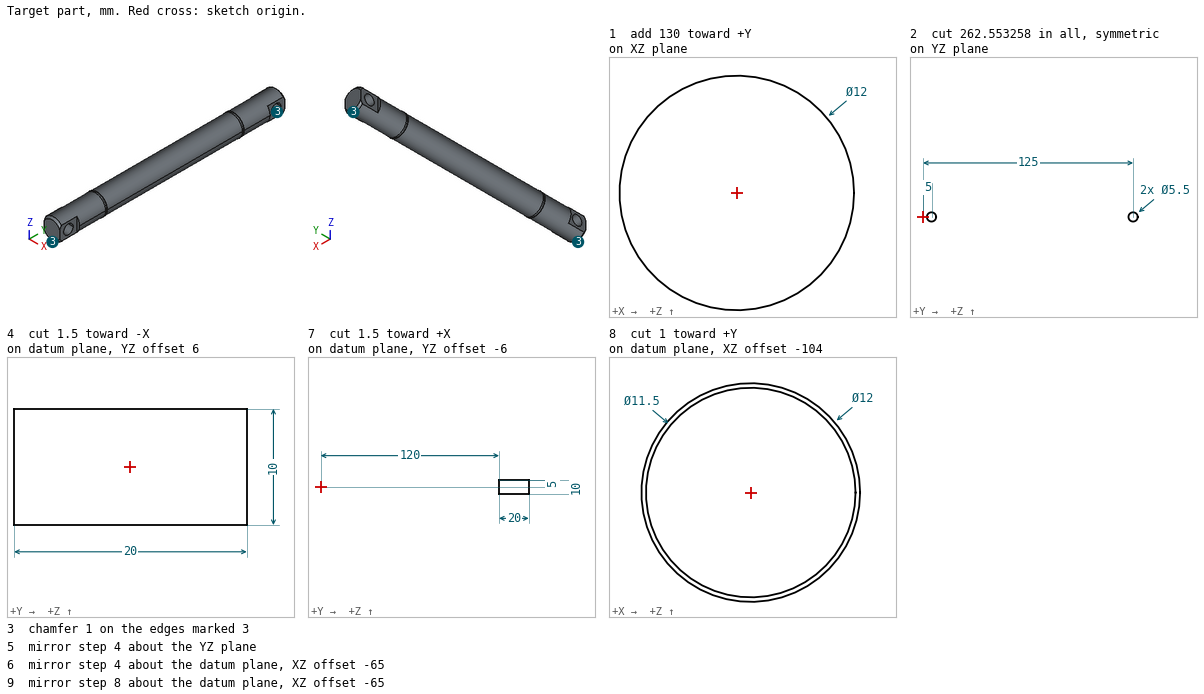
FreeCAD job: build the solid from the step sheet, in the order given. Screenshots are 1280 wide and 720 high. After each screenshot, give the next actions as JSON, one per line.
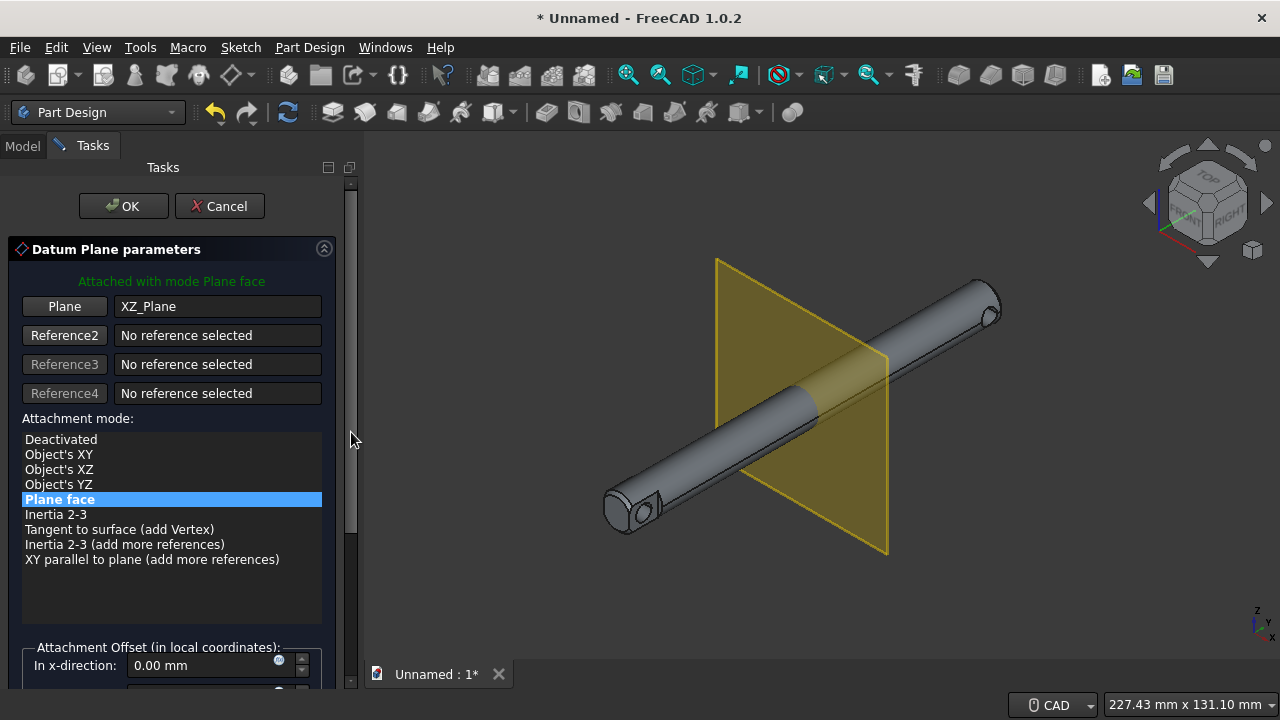
{"action": "left_click", "coordinate": [124, 206]}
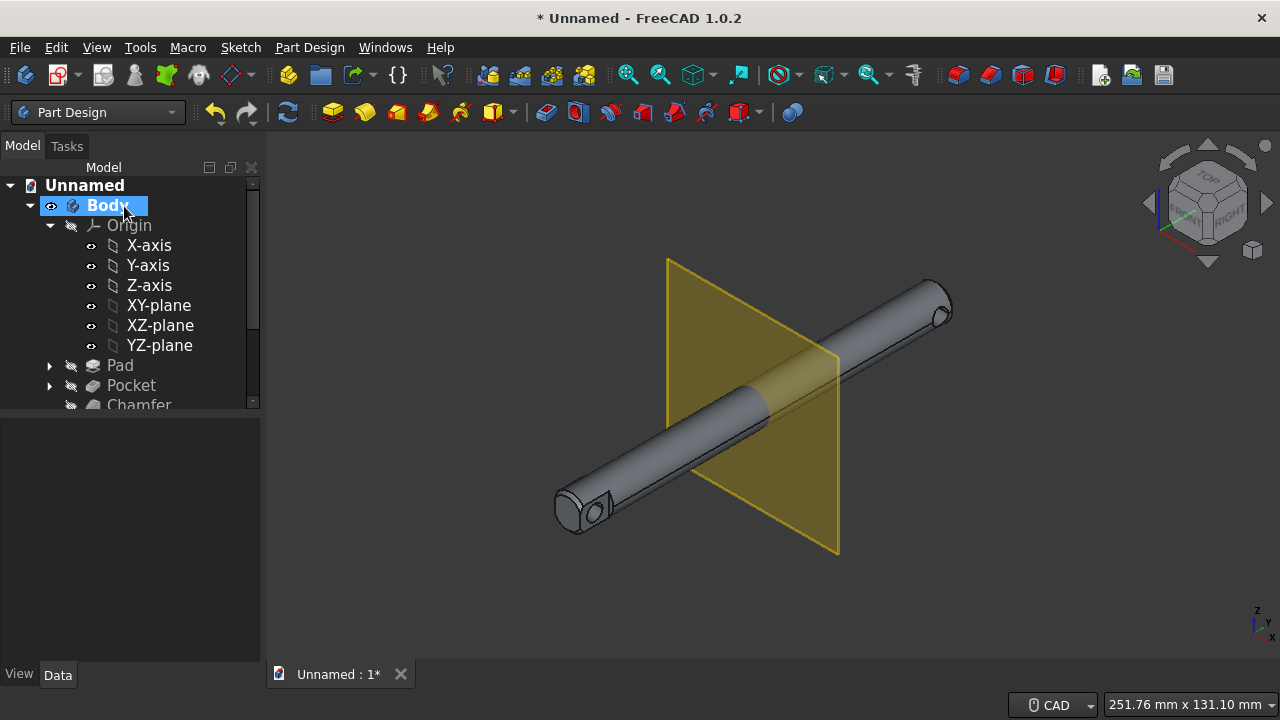
{"action": "scroll", "coordinate": [100, 301], "scroll_direction": "down", "scroll_amount": 3}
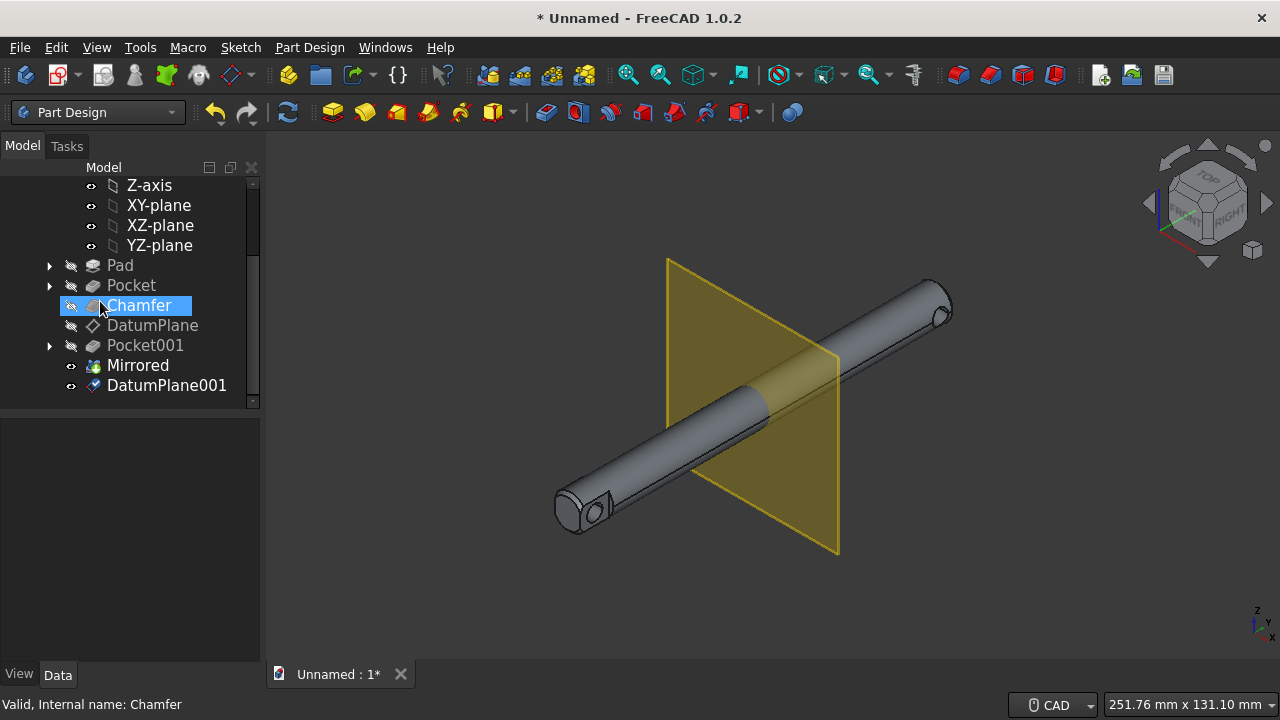
{"action": "left_click", "coordinate": [116, 346]}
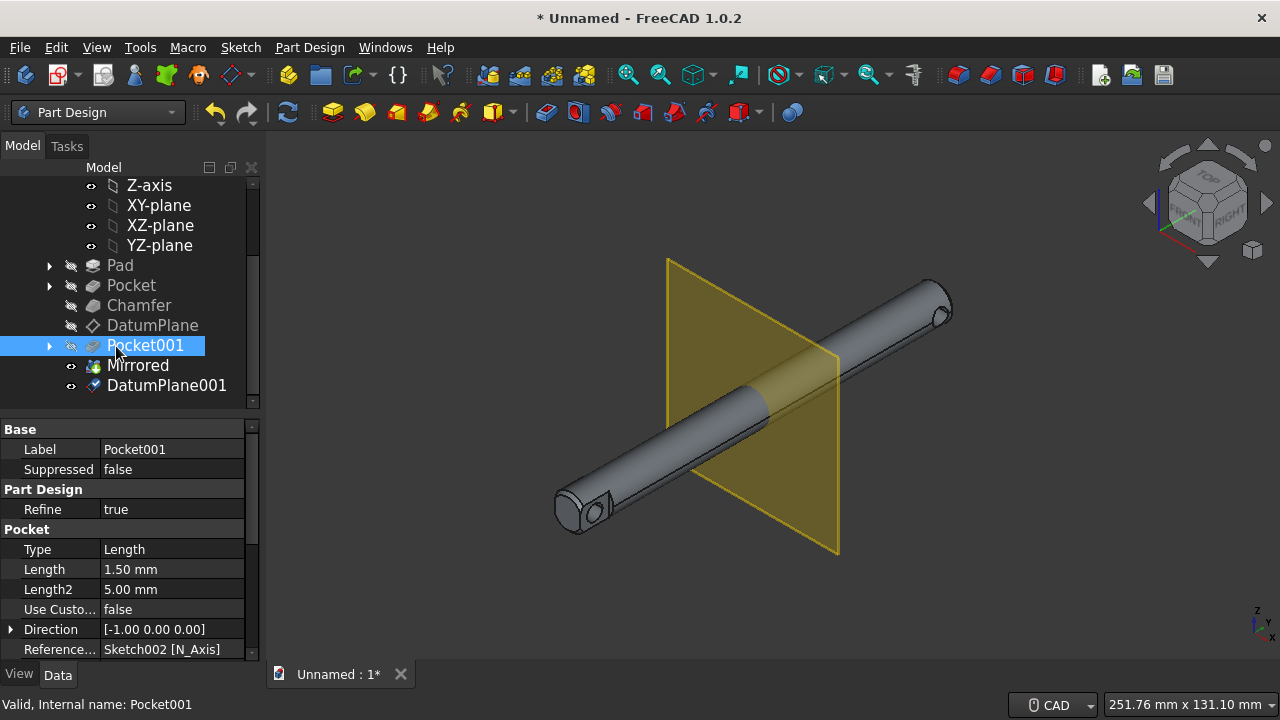
{"action": "left_click", "coordinate": [488, 76]}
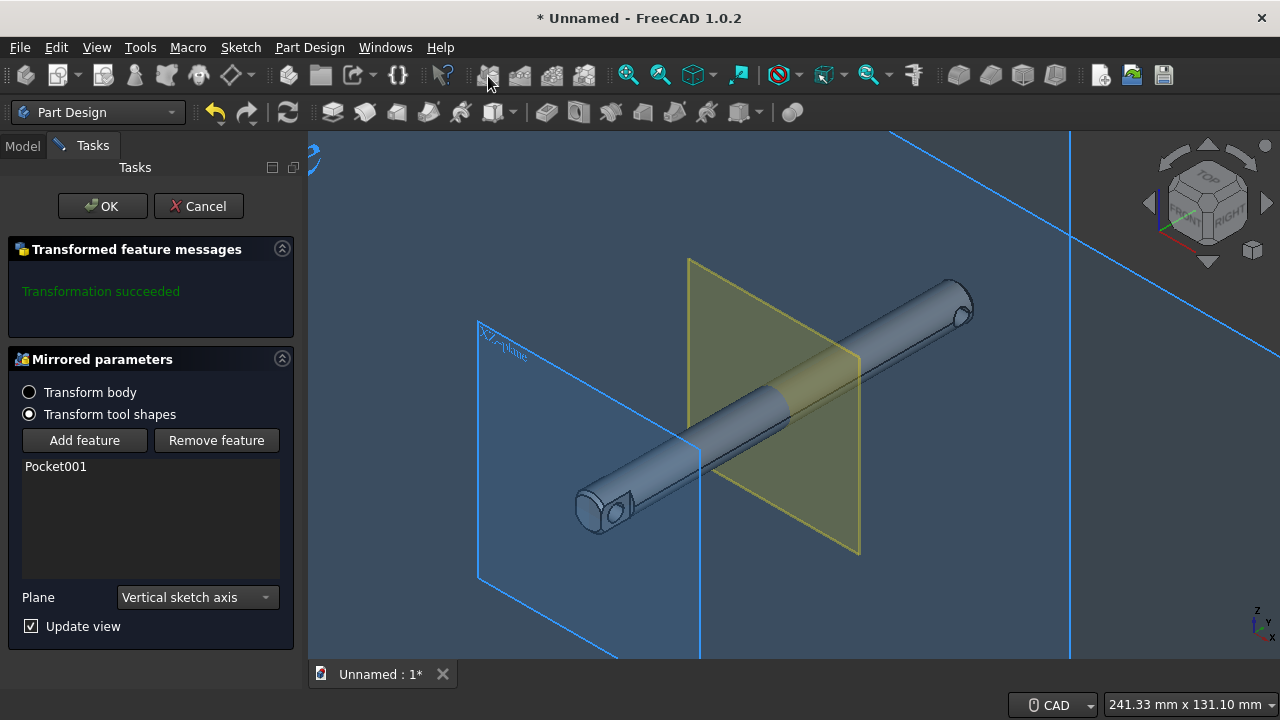
{"action": "left_click", "coordinate": [198, 598]}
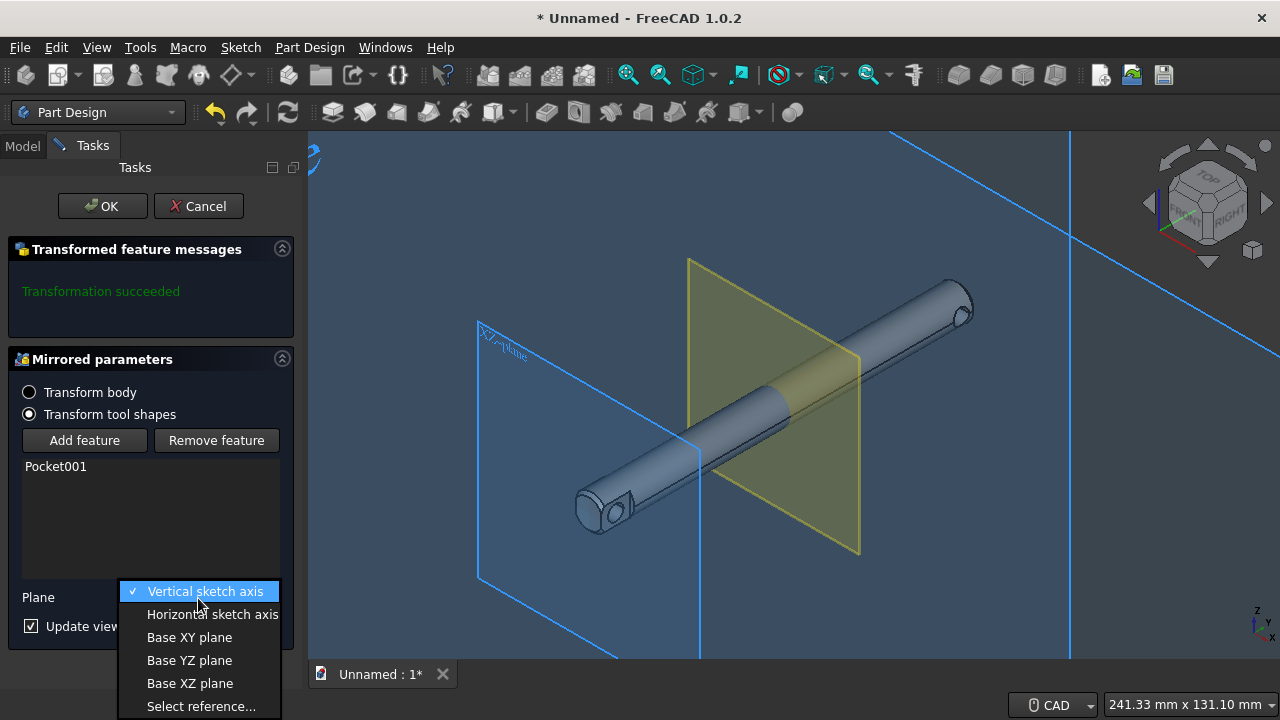
{"action": "left_click", "coordinate": [198, 706]}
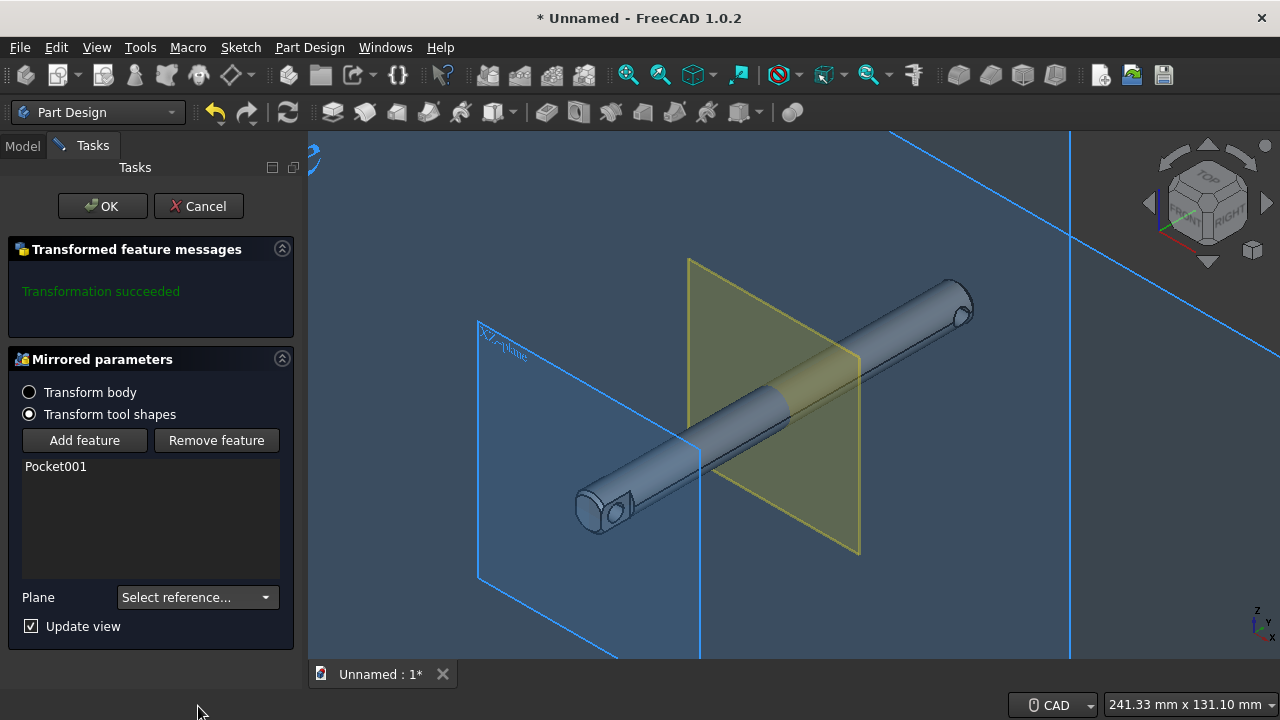
{"action": "left_click", "coordinate": [23, 145]}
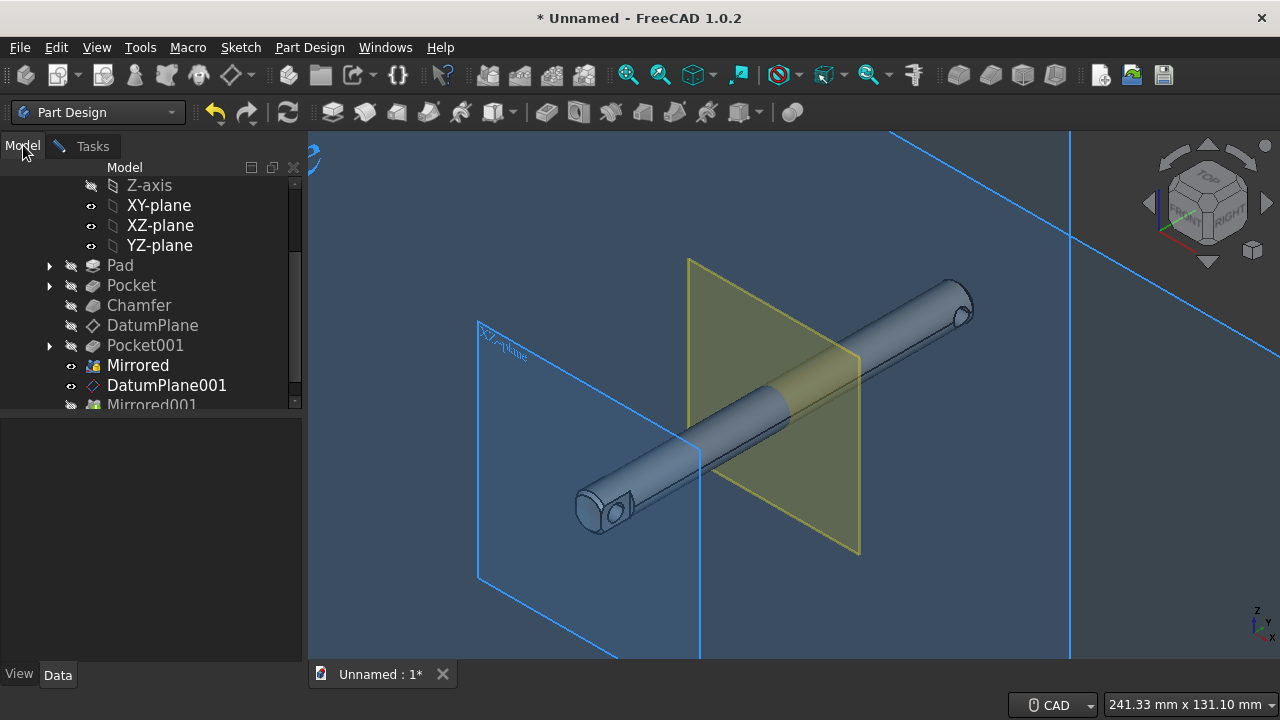
{"action": "left_click", "coordinate": [116, 386]}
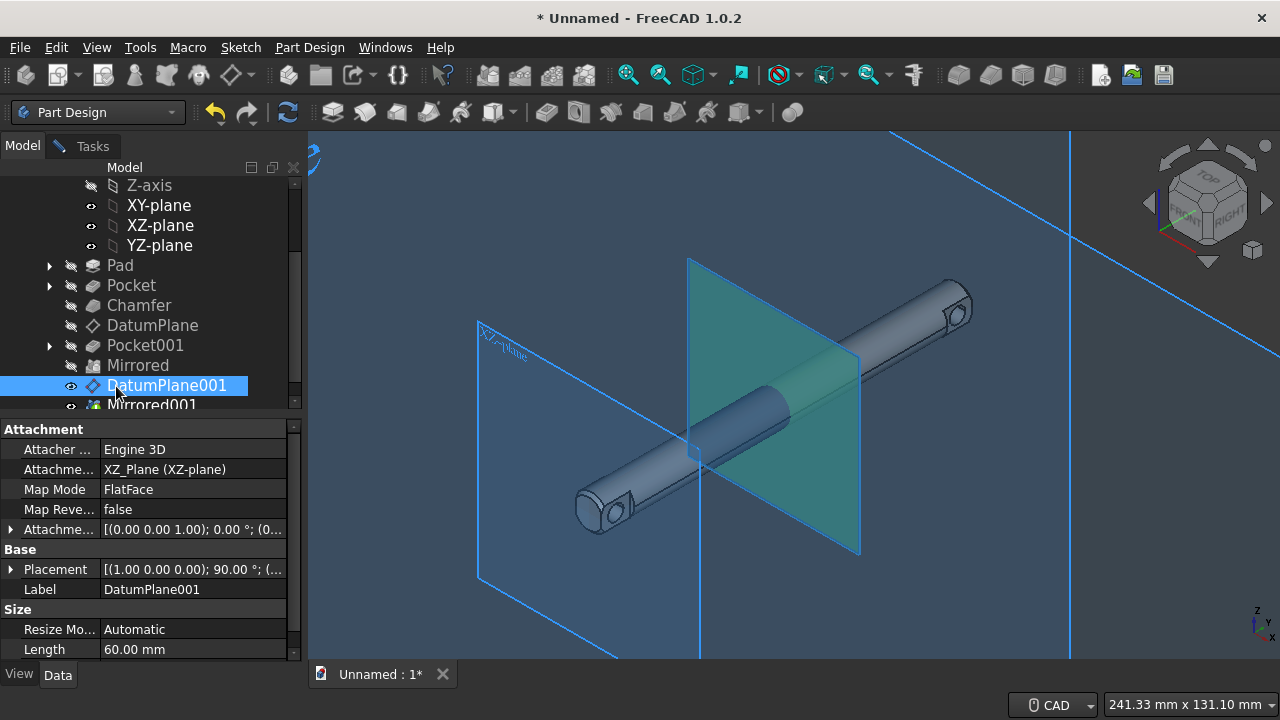
{"action": "left_click", "coordinate": [84, 145]}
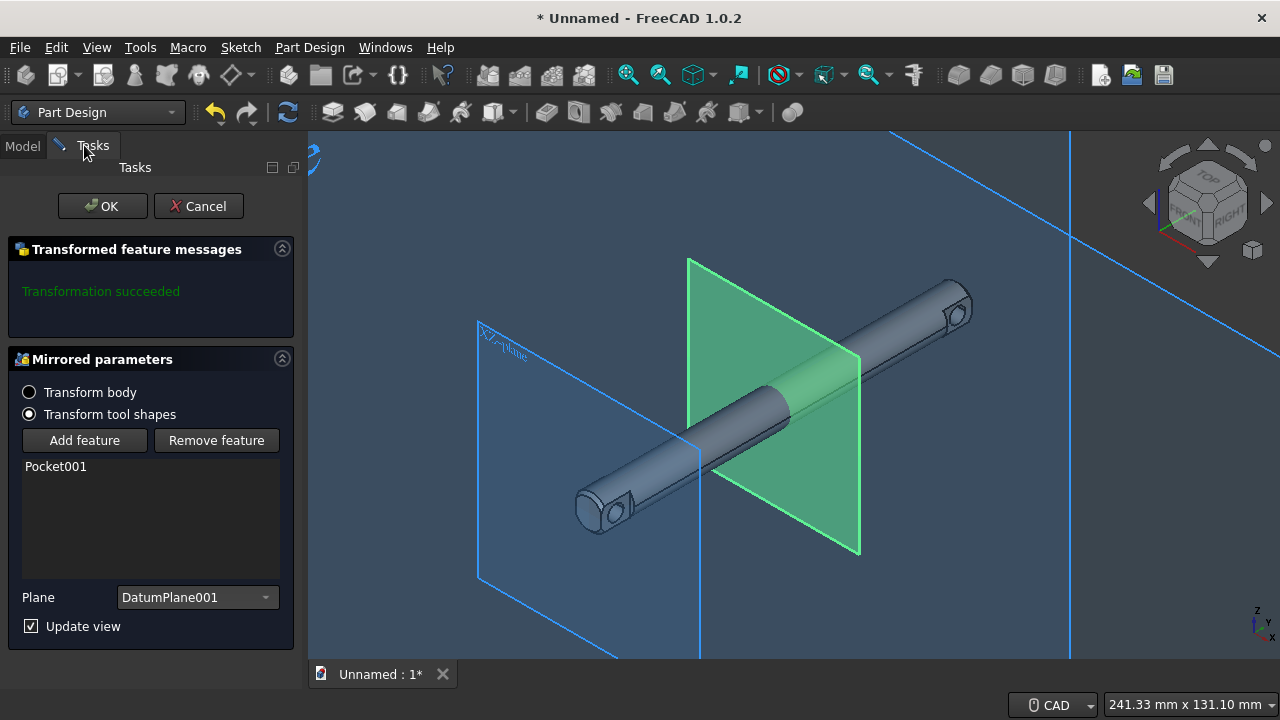
{"action": "left_click", "coordinate": [103, 206]}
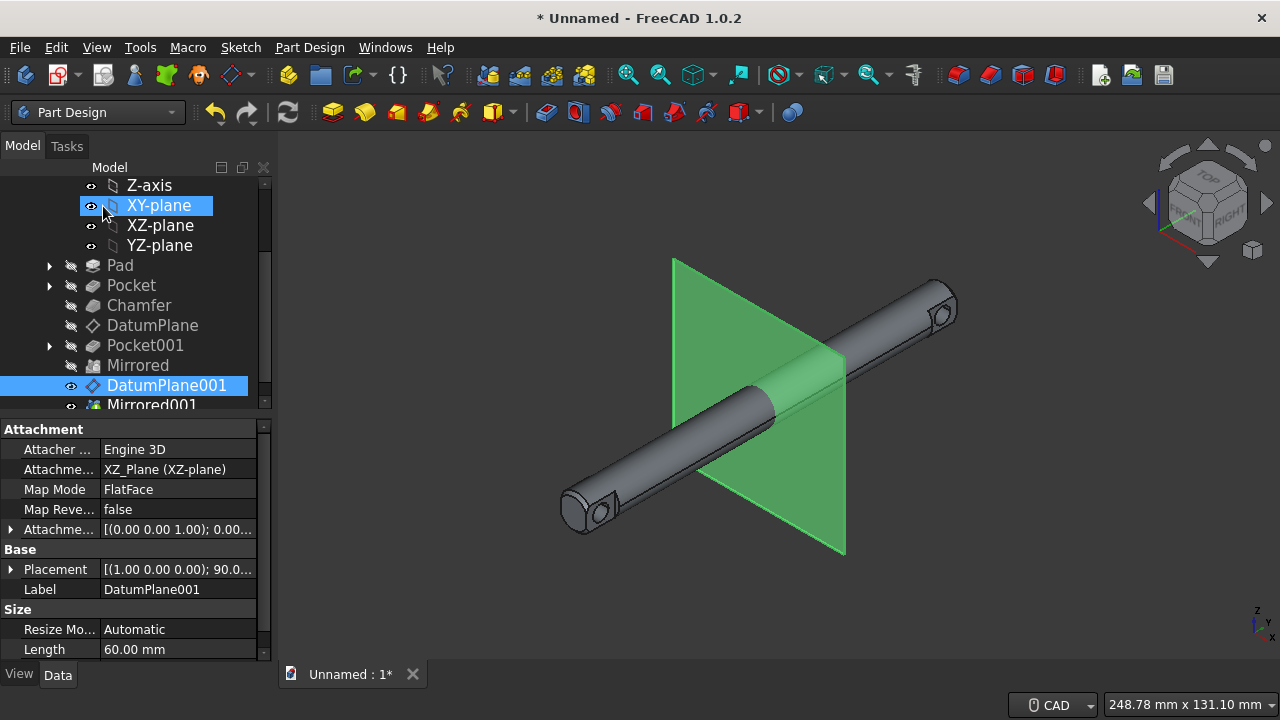
{"action": "left_click", "coordinate": [116, 386]}
{"action": "key", "text": "space"}